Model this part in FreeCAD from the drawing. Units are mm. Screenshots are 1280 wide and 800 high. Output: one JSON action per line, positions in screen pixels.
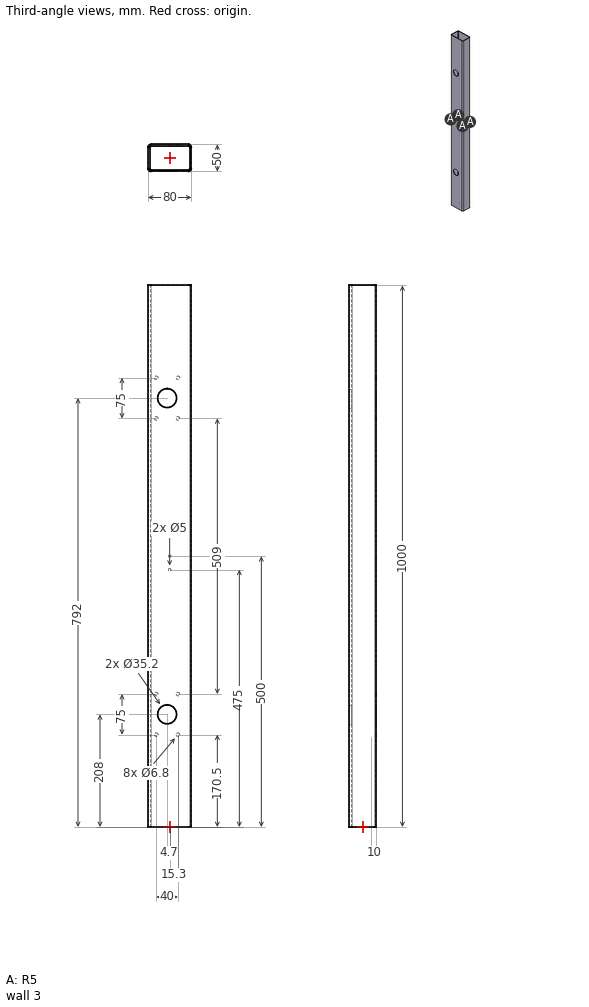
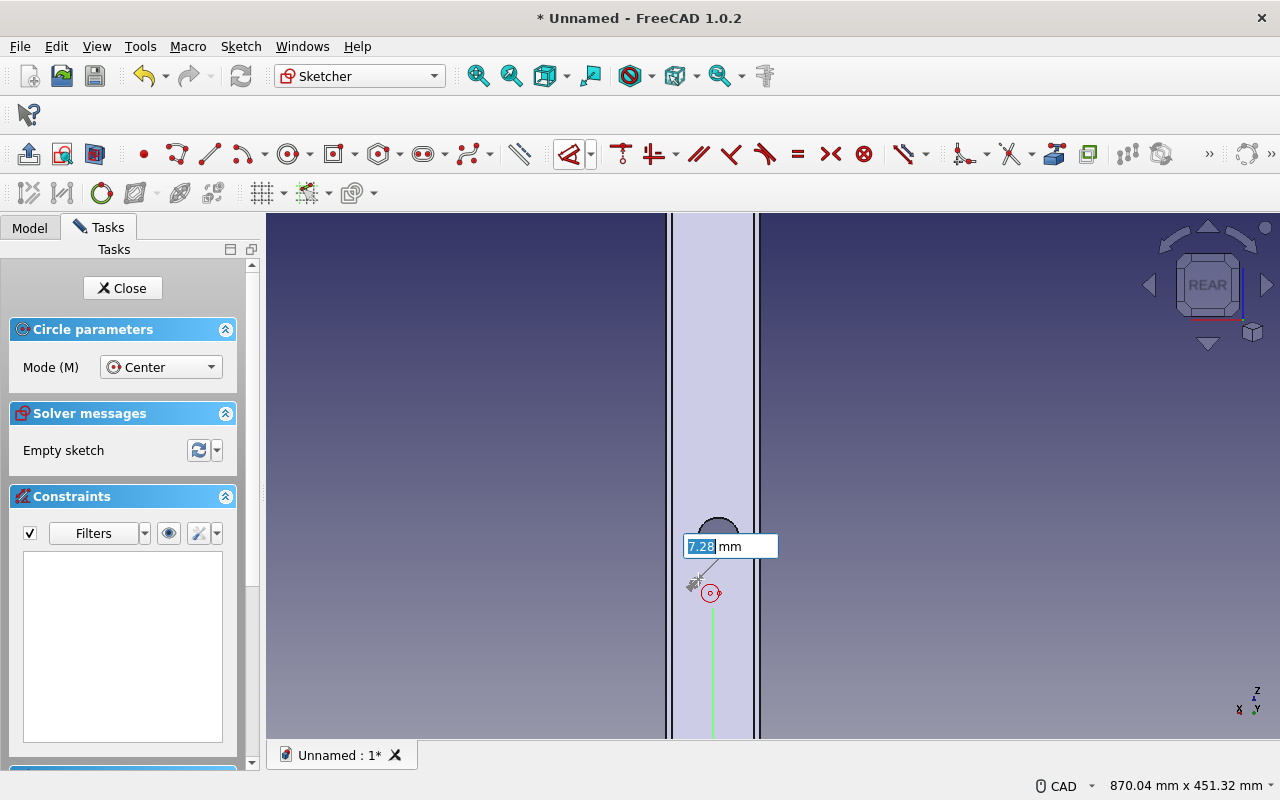
{"action": "type", "text": "6.8"}
{"action": "key", "text": "Return"}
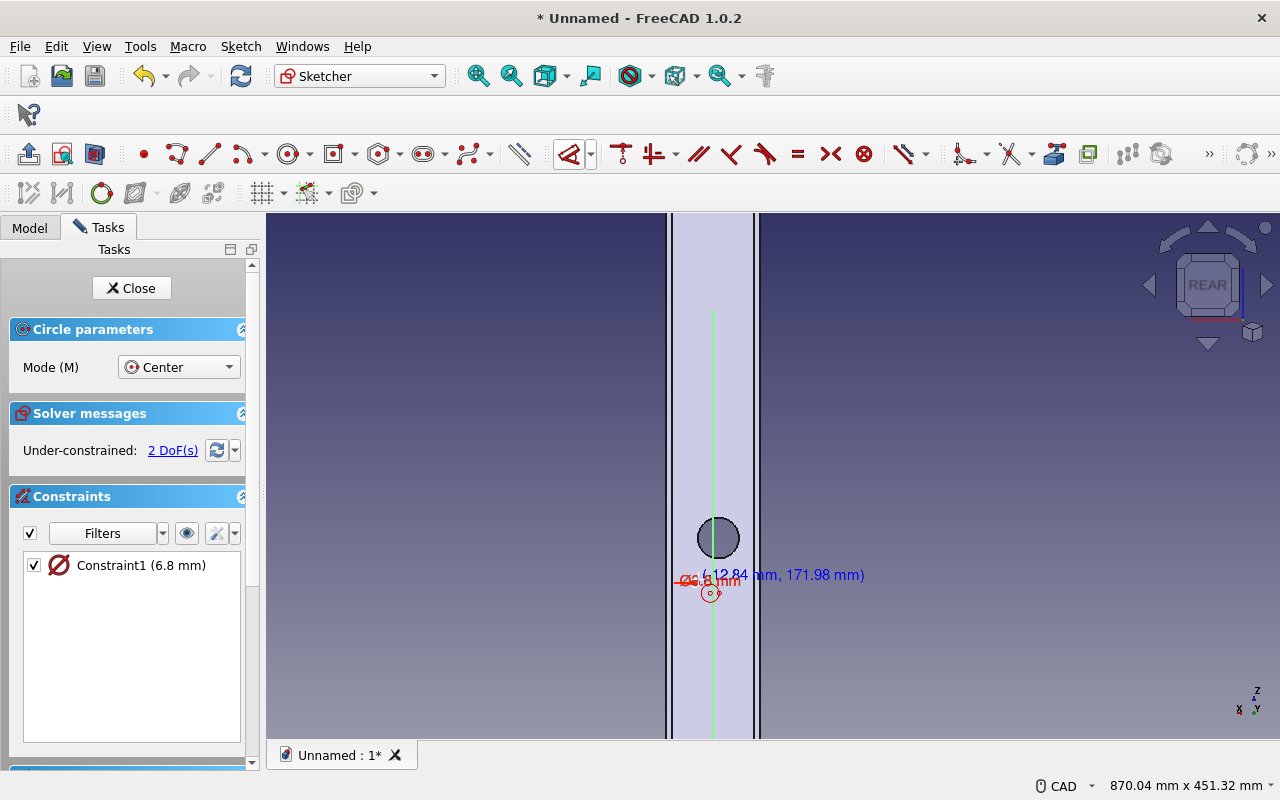
{"action": "scroll", "coordinate": [742, 582], "scroll_direction": "up", "scroll_amount": 9}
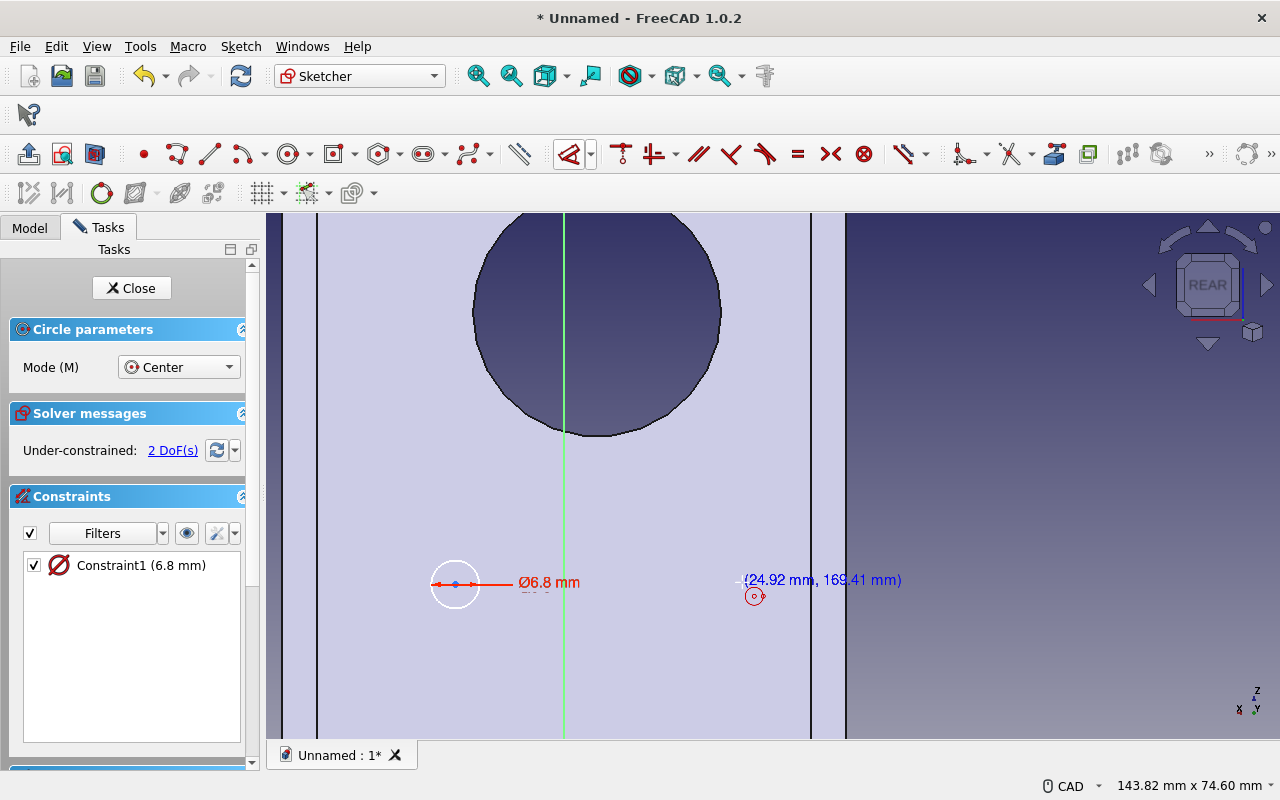
{"action": "scroll", "coordinate": [711, 582], "scroll_direction": "down", "scroll_amount": 14}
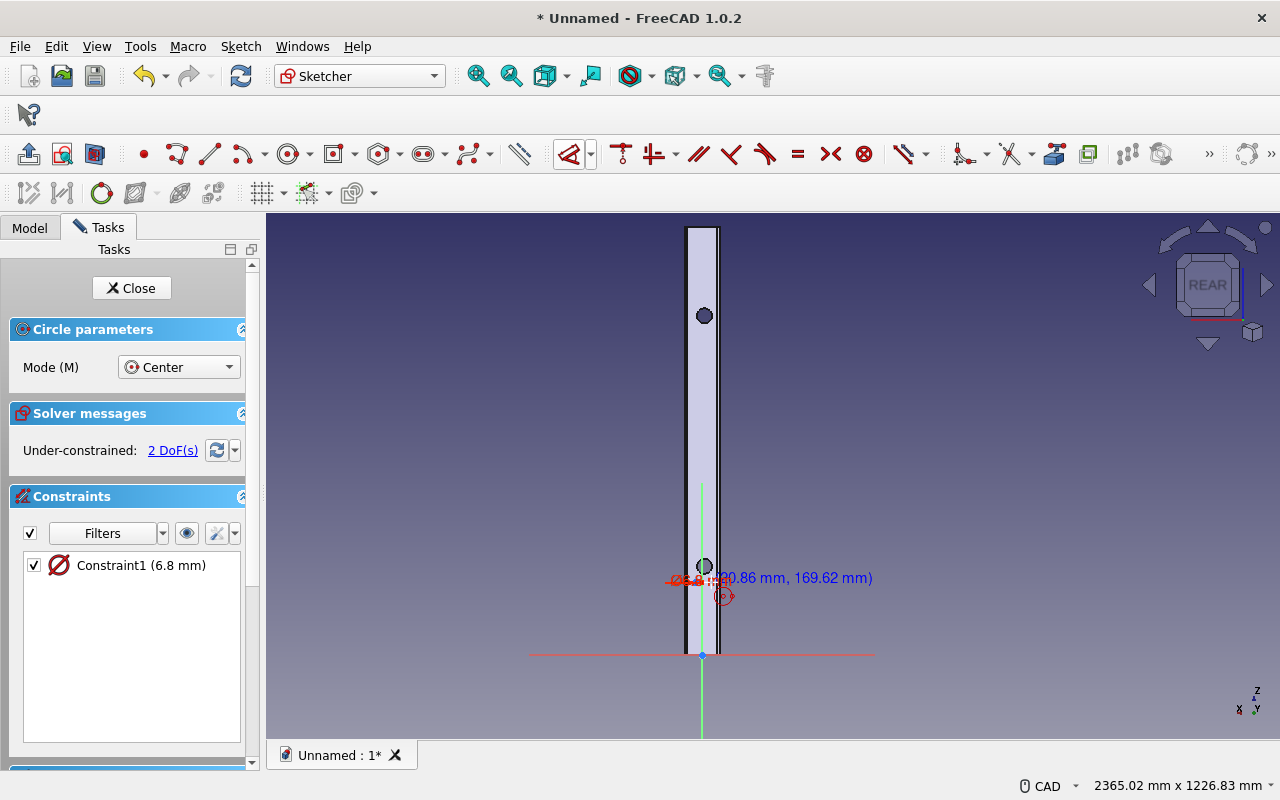
{"action": "scroll", "coordinate": [713, 582], "scroll_direction": "up", "scroll_amount": 3}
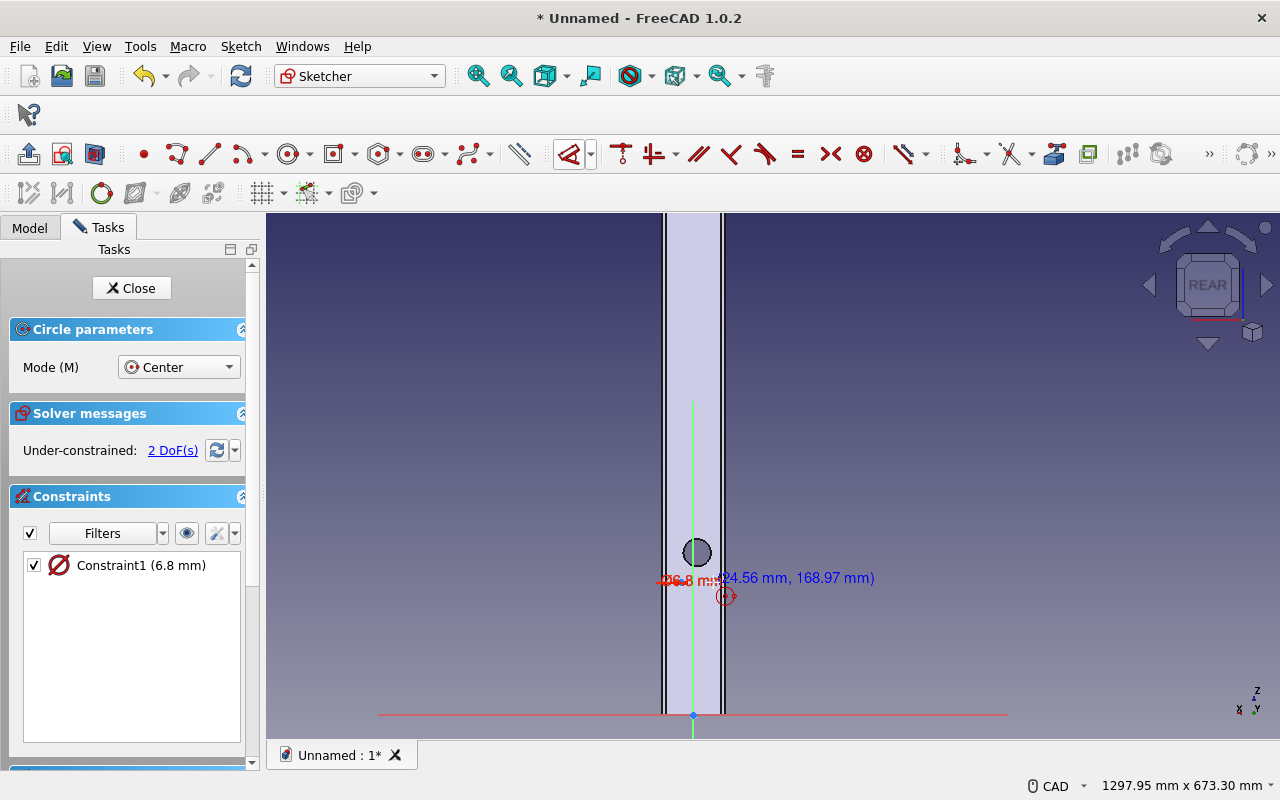
{"action": "left_click", "coordinate": [713, 582]}
{"action": "mouse_move", "coordinate": [715, 580]}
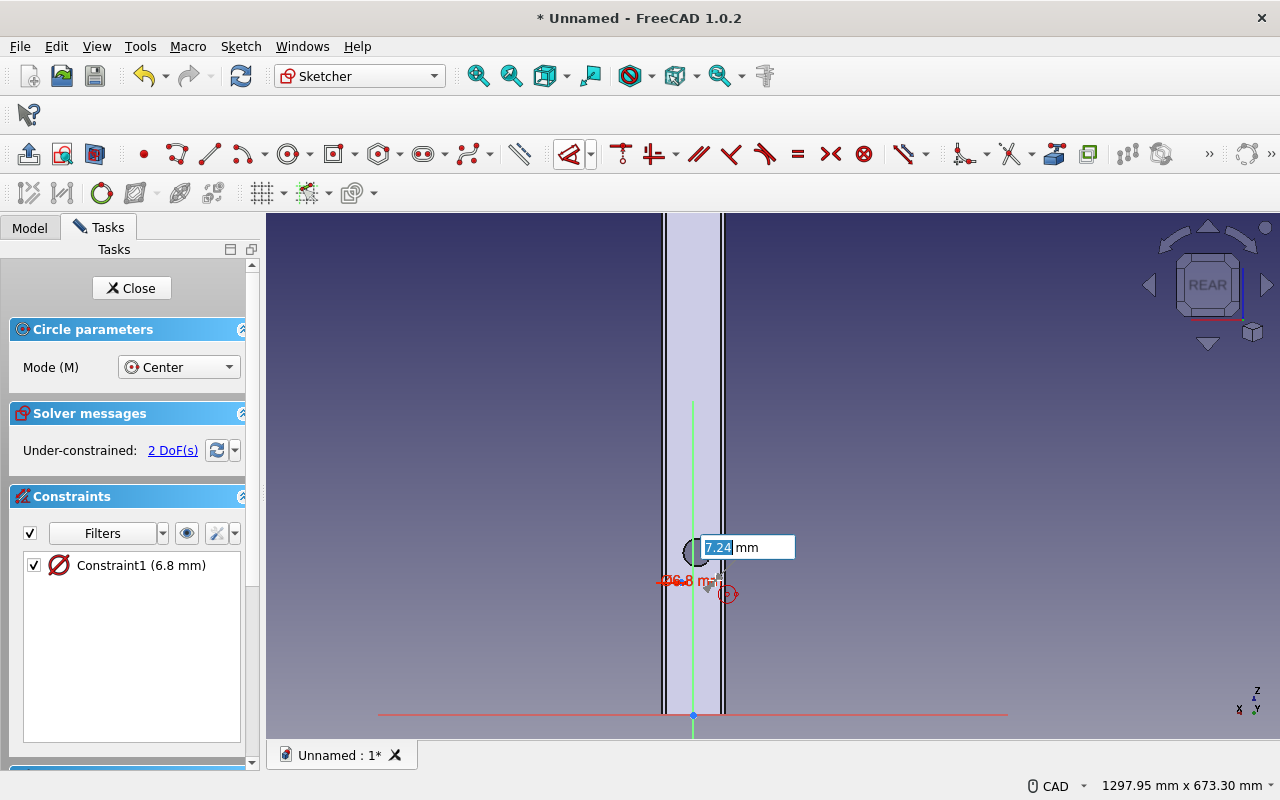
{"action": "type", "text": "6.8"}
{"action": "key", "text": "Return"}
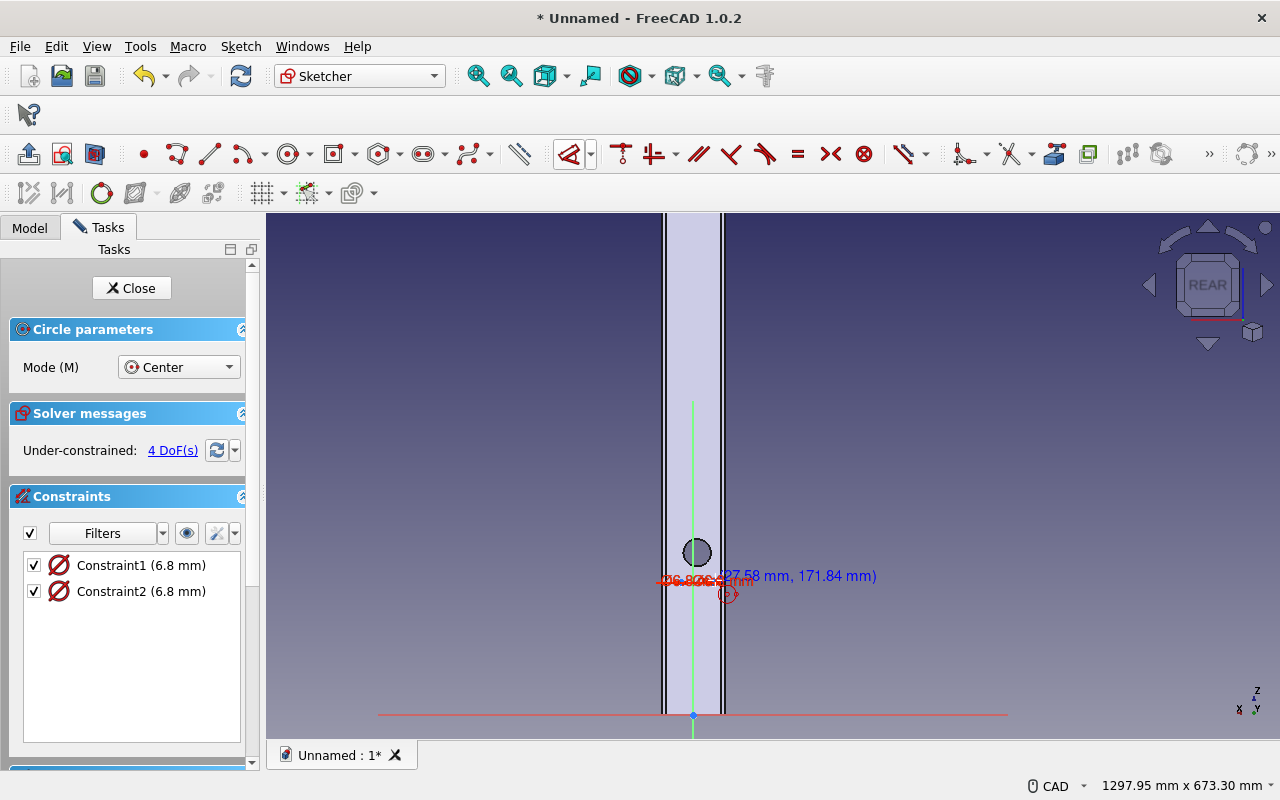
{"action": "scroll", "coordinate": [713, 523], "scroll_direction": "up", "scroll_amount": 11}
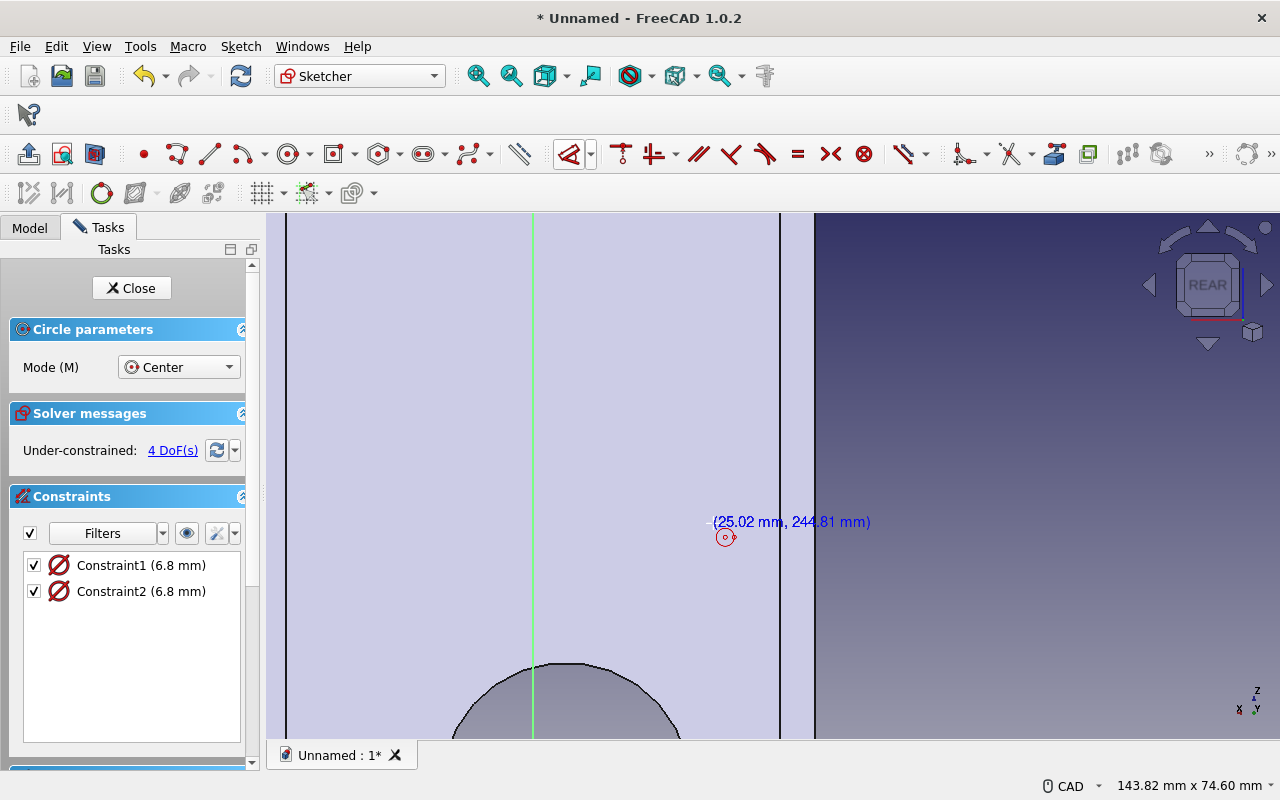
{"action": "scroll", "coordinate": [713, 551], "scroll_direction": "down", "scroll_amount": 14}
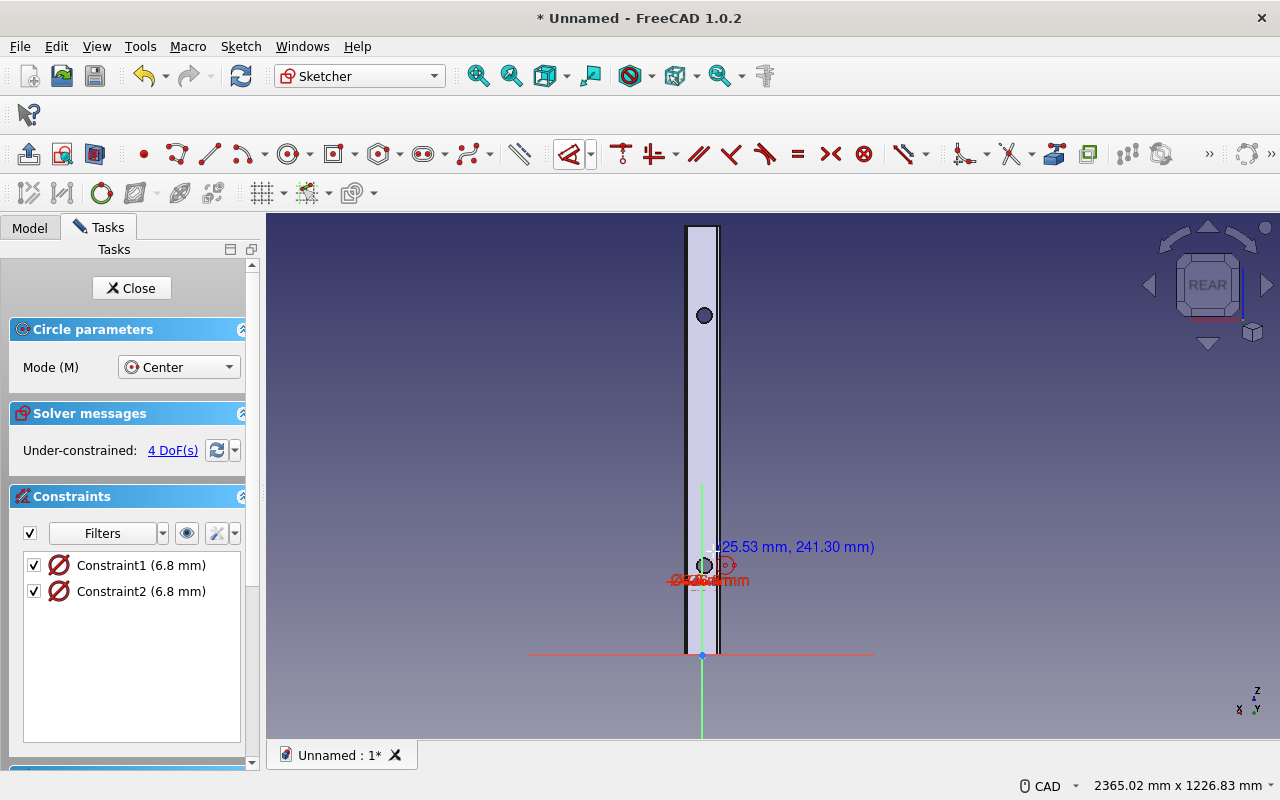
{"action": "scroll", "coordinate": [713, 550], "scroll_direction": "up", "scroll_amount": 3}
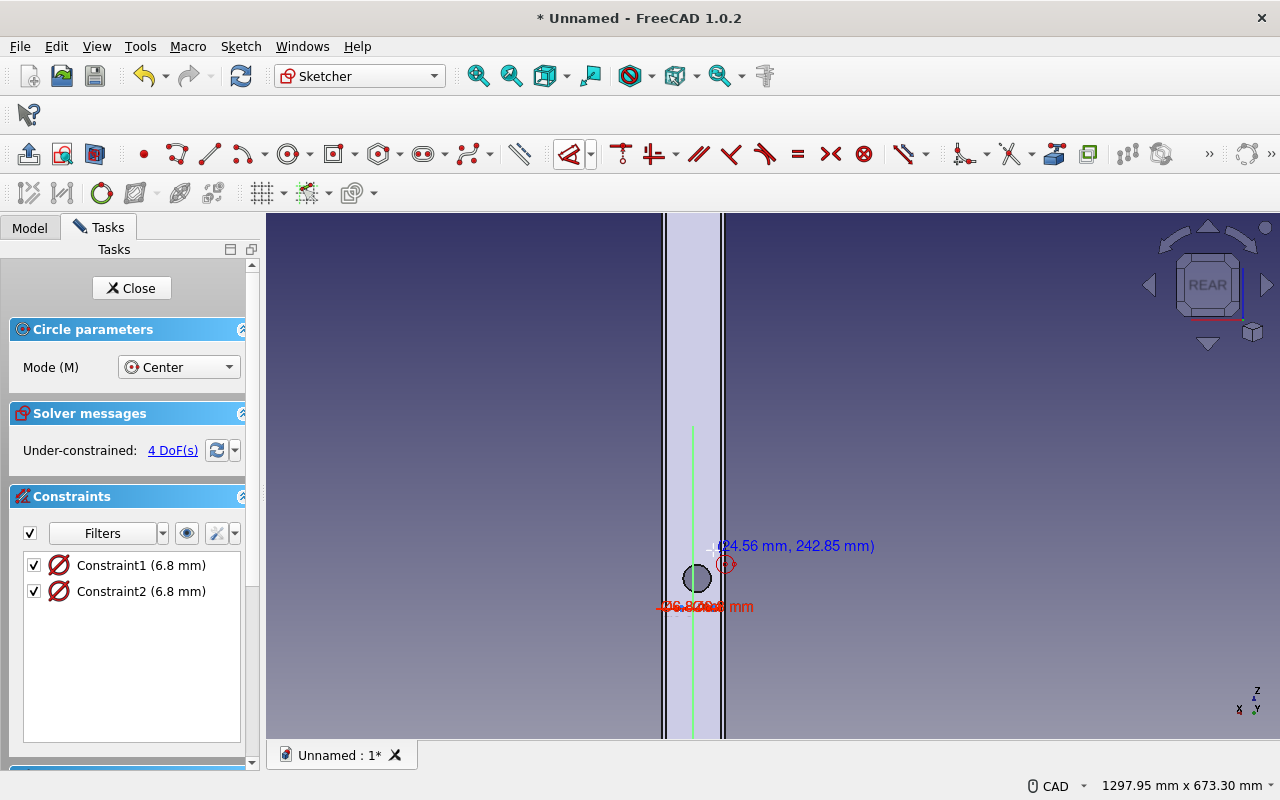
{"action": "left_click", "coordinate": [713, 549]}
{"action": "mouse_move", "coordinate": [715, 547]}